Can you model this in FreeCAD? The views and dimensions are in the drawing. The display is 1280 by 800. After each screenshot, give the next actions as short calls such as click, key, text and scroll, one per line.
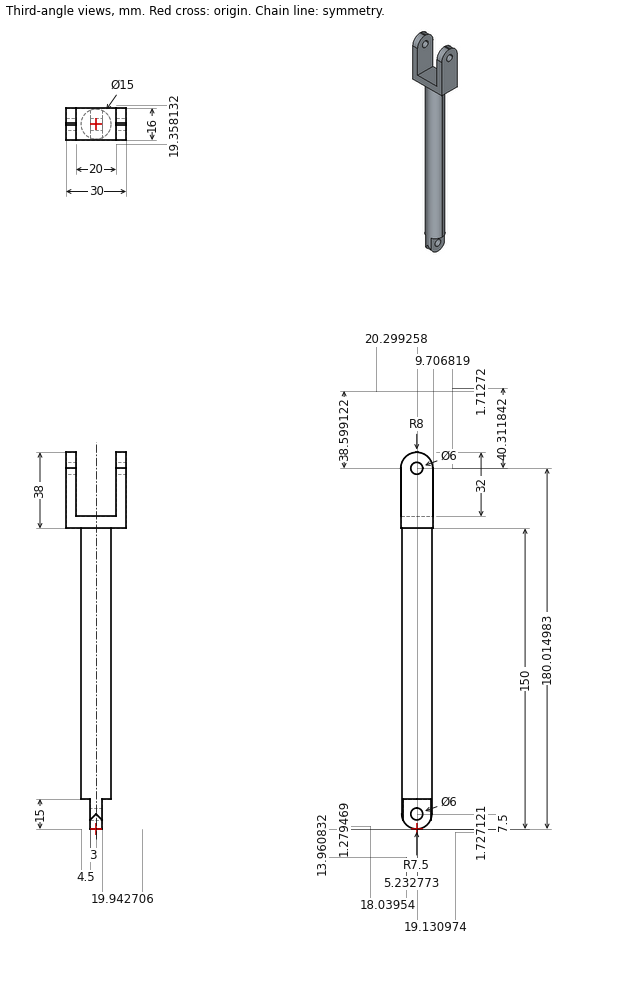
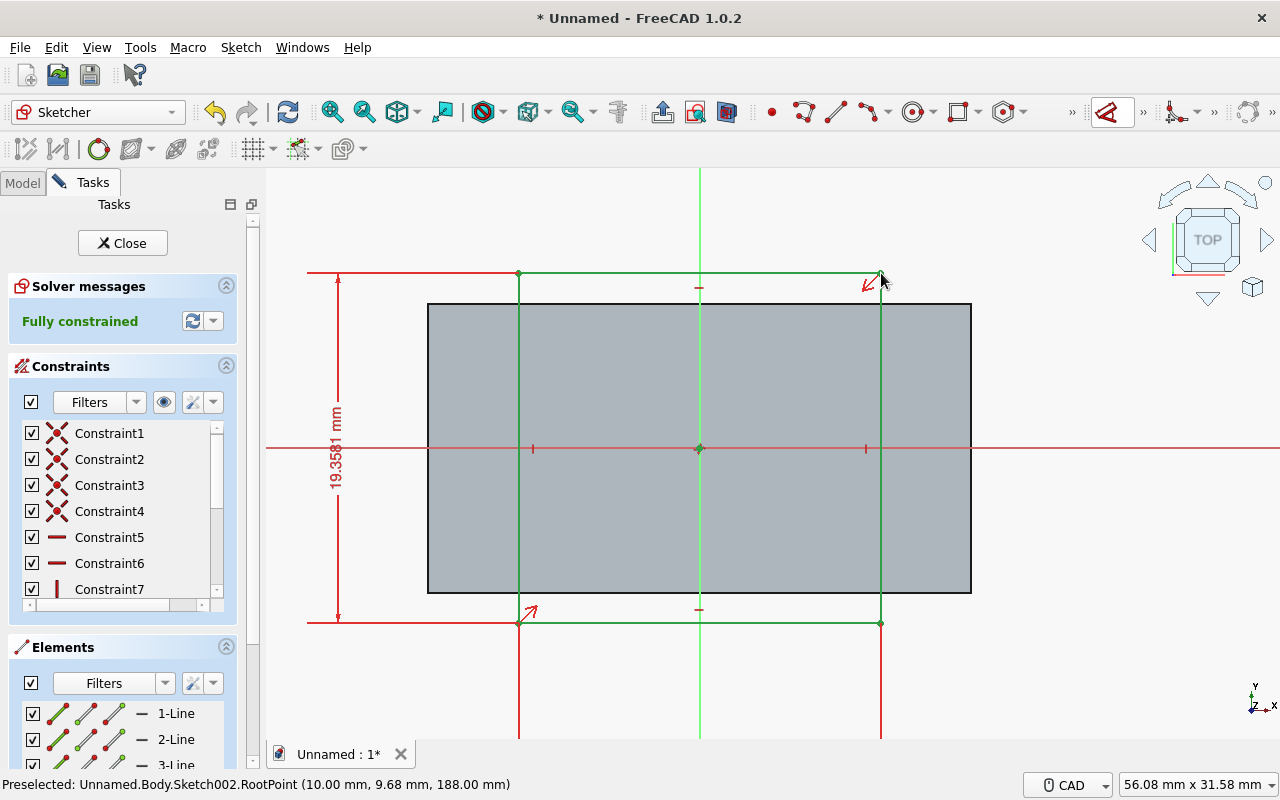
click(123, 243)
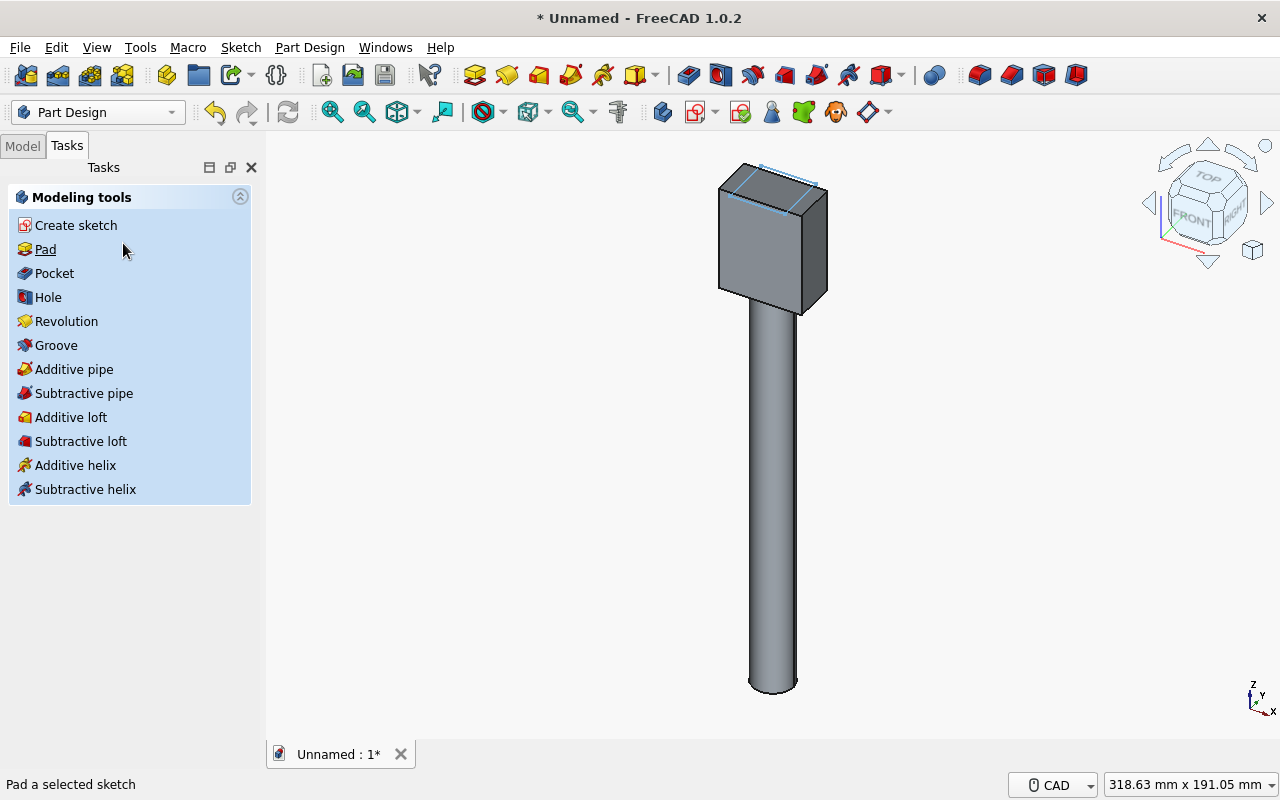
click(690, 76)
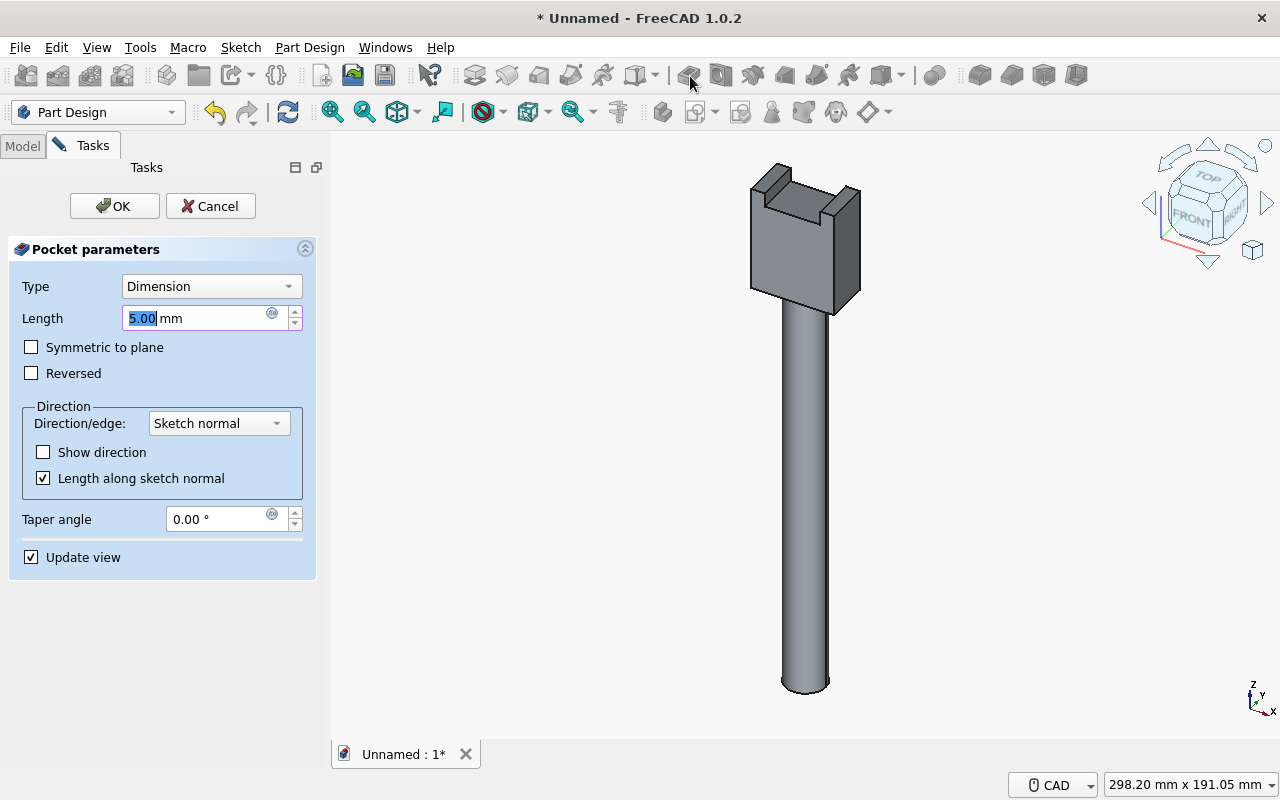
text(32)
key(Tab)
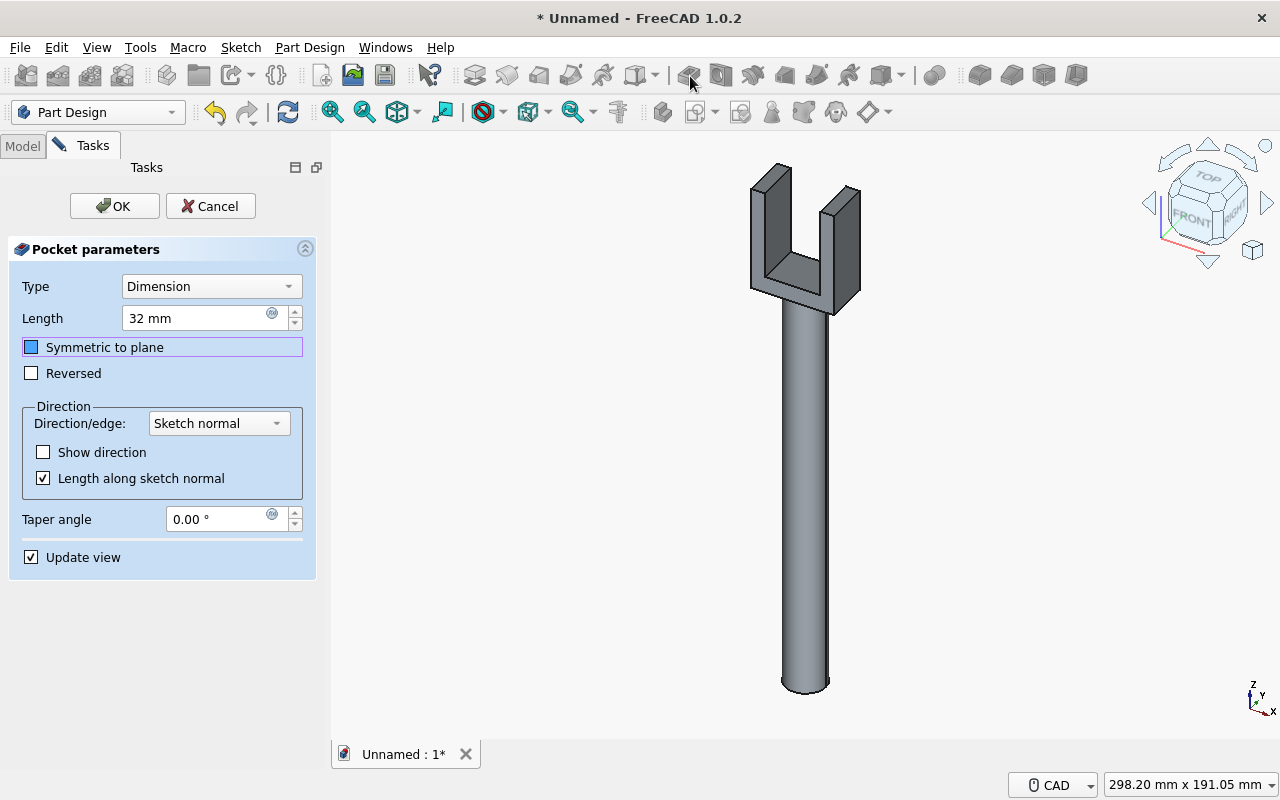
click(115, 206)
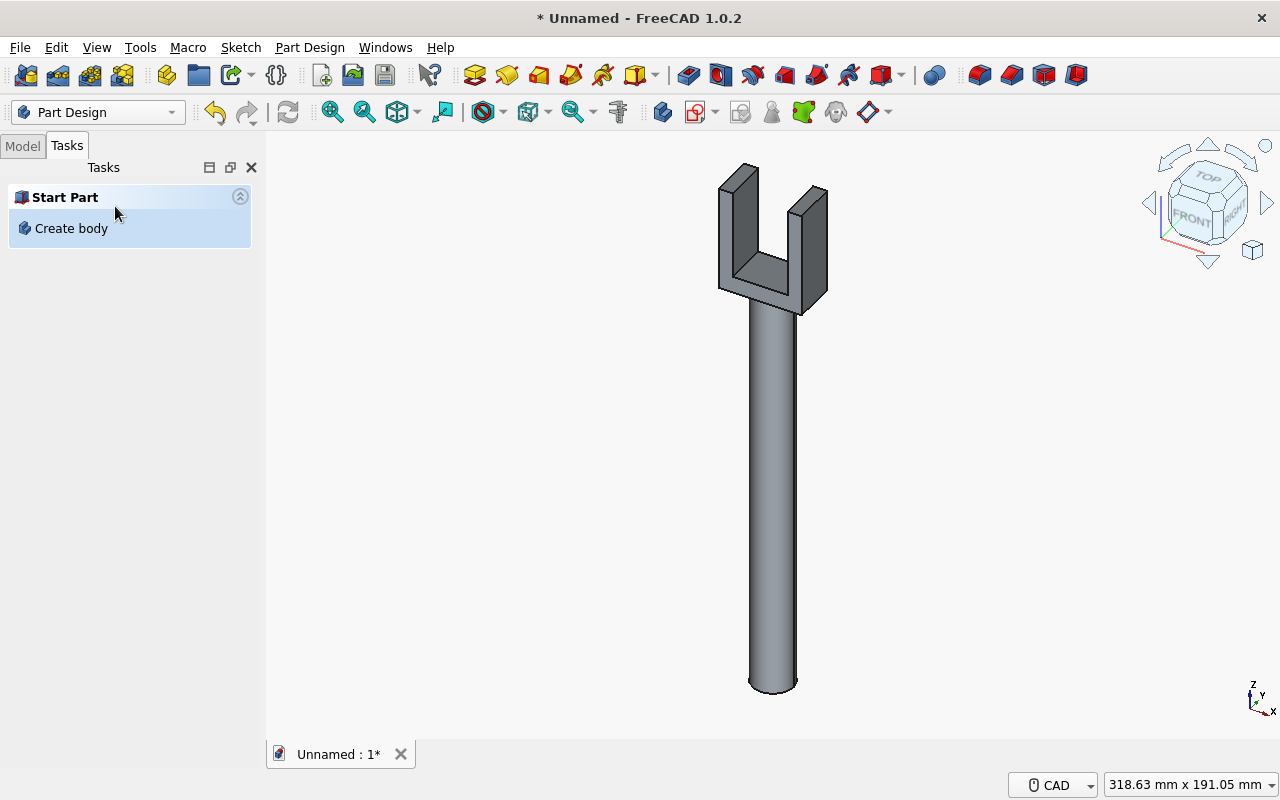
click(814, 224)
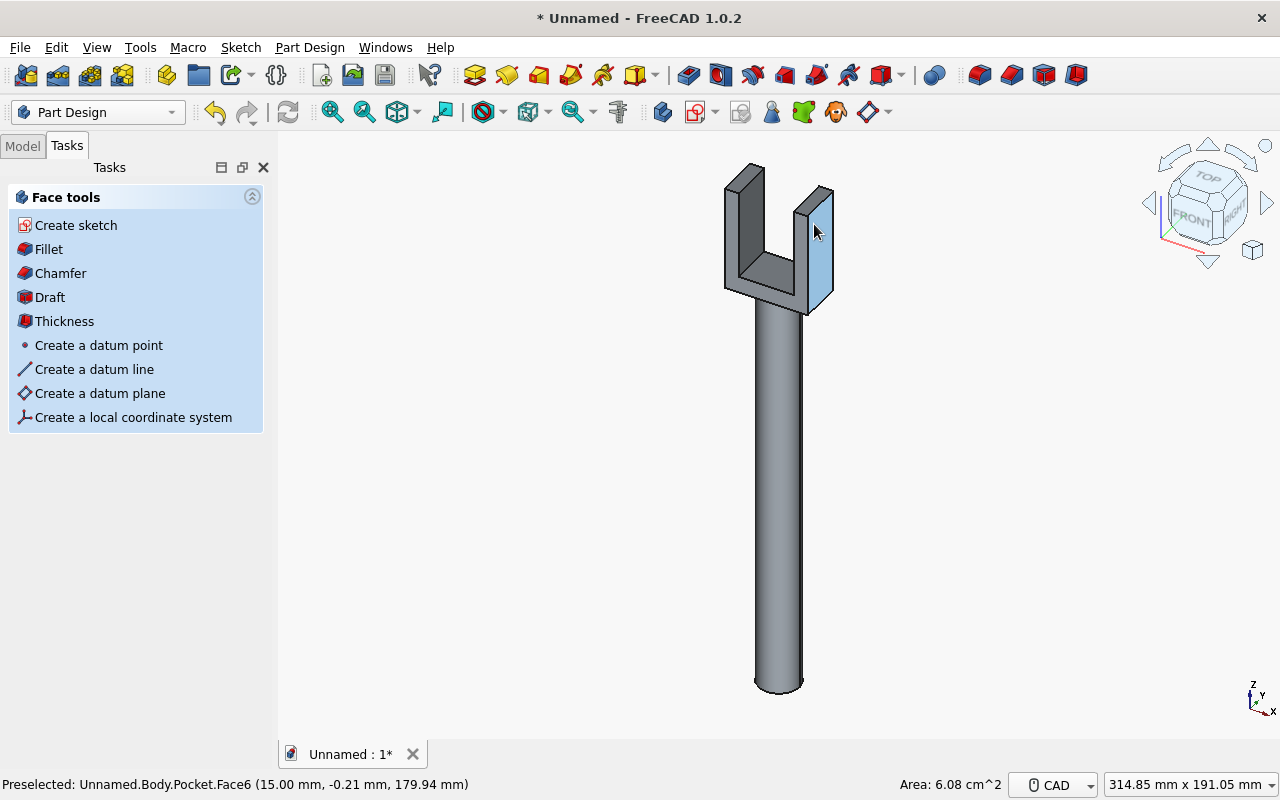
click(696, 112)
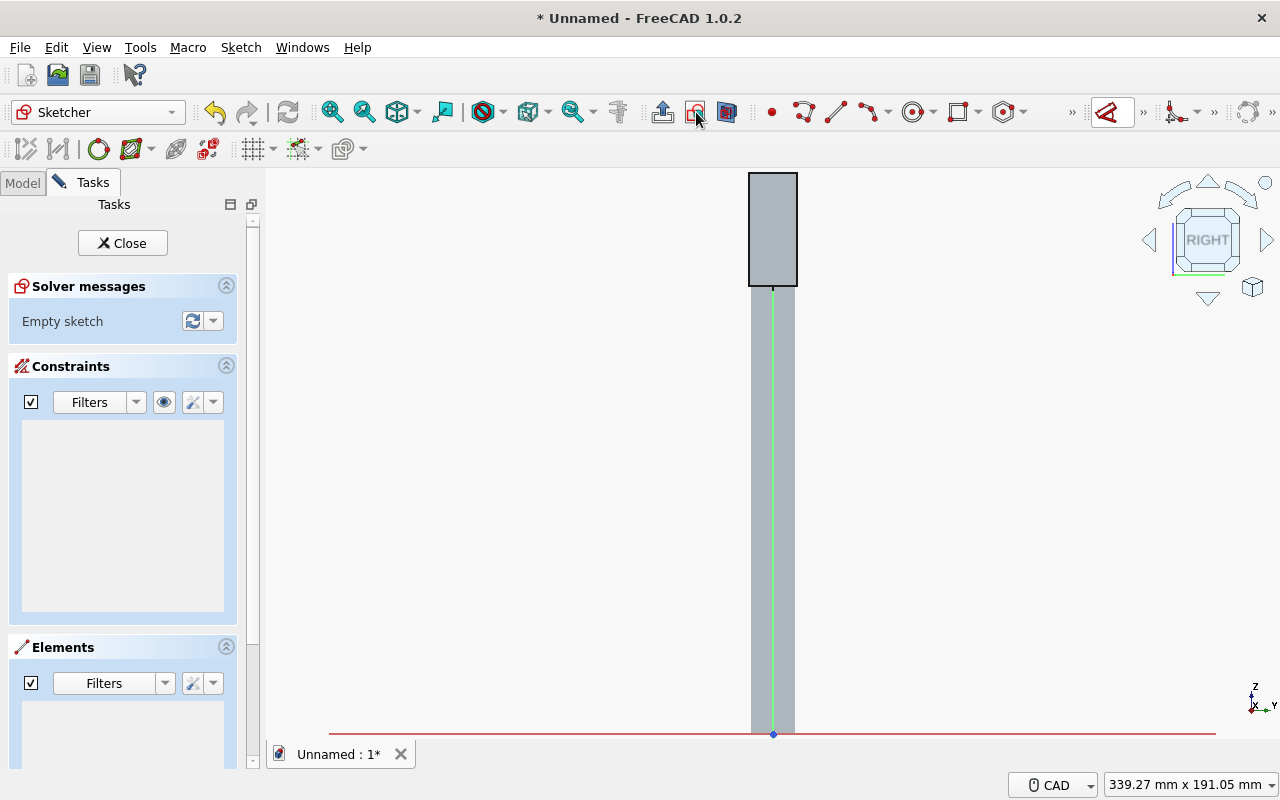
scroll(704, 454, down, 5)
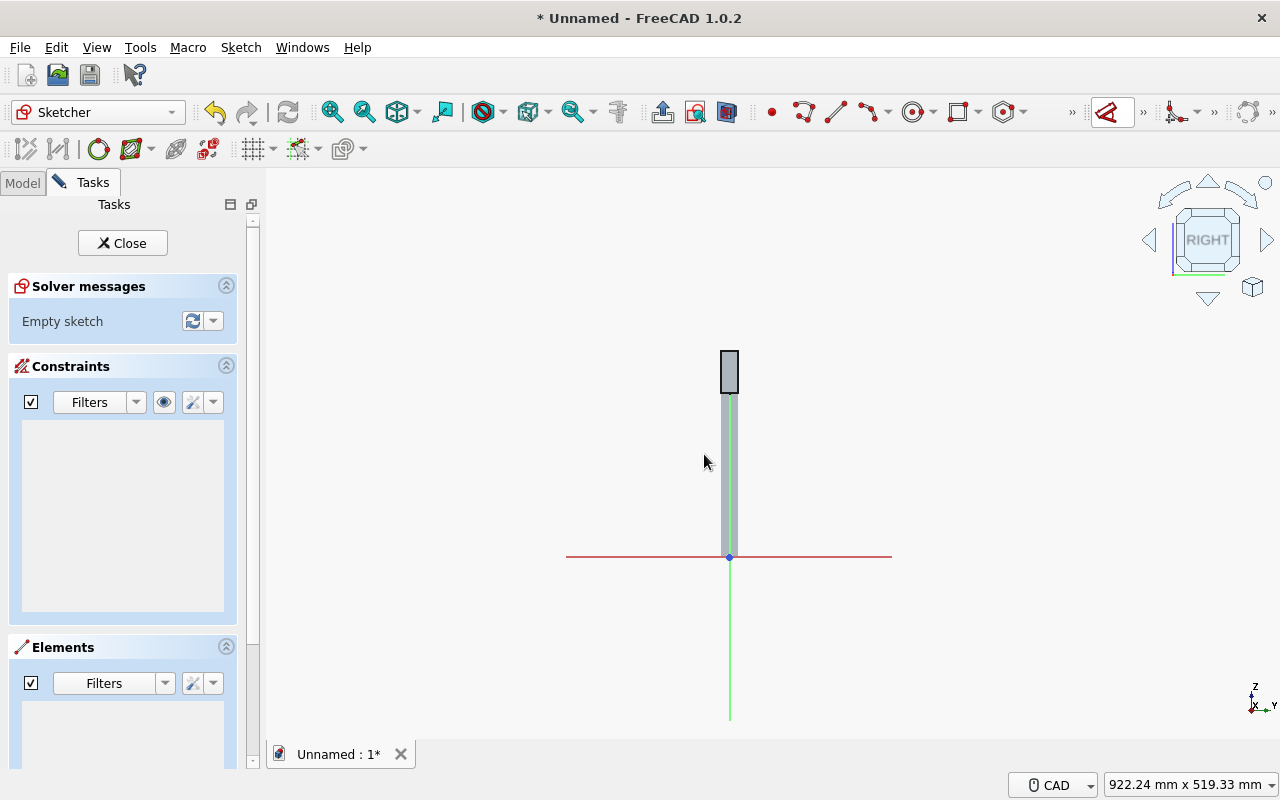
scroll(732, 321, up, 10)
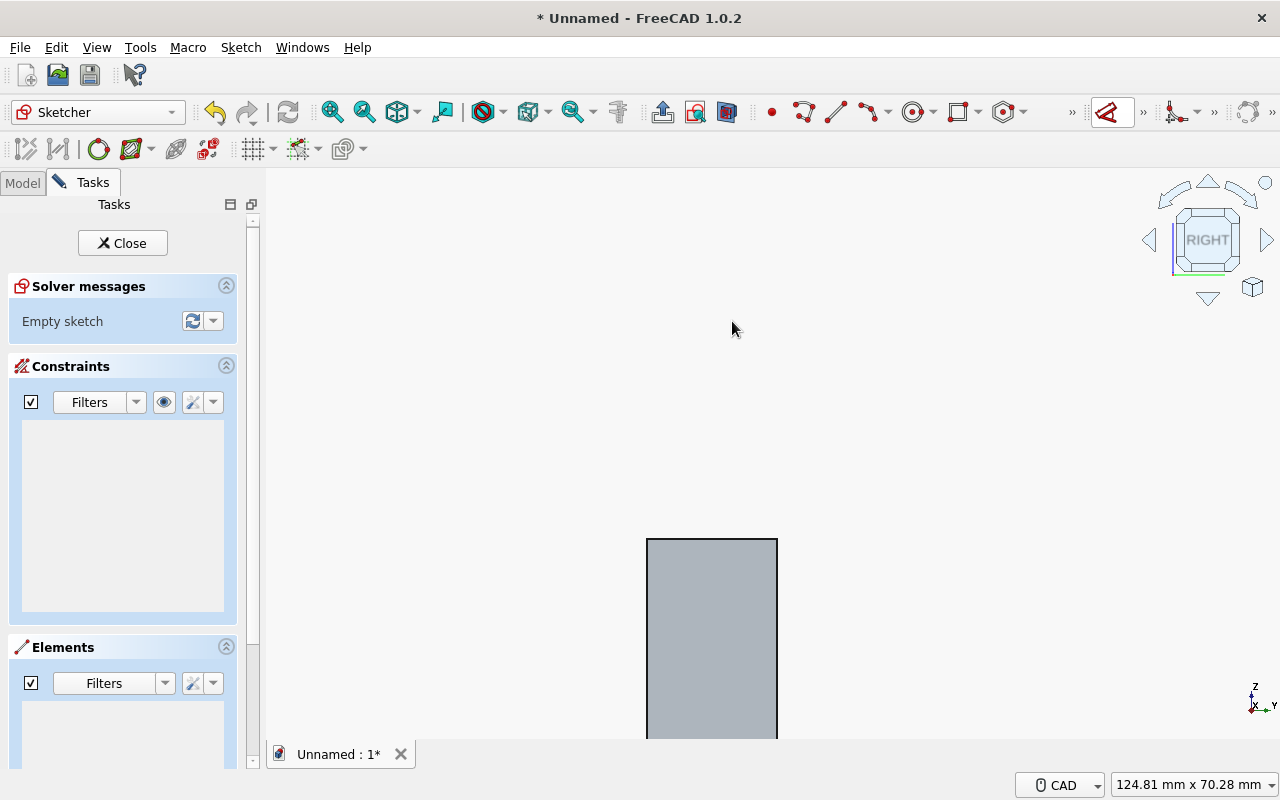
key(g)
key(m)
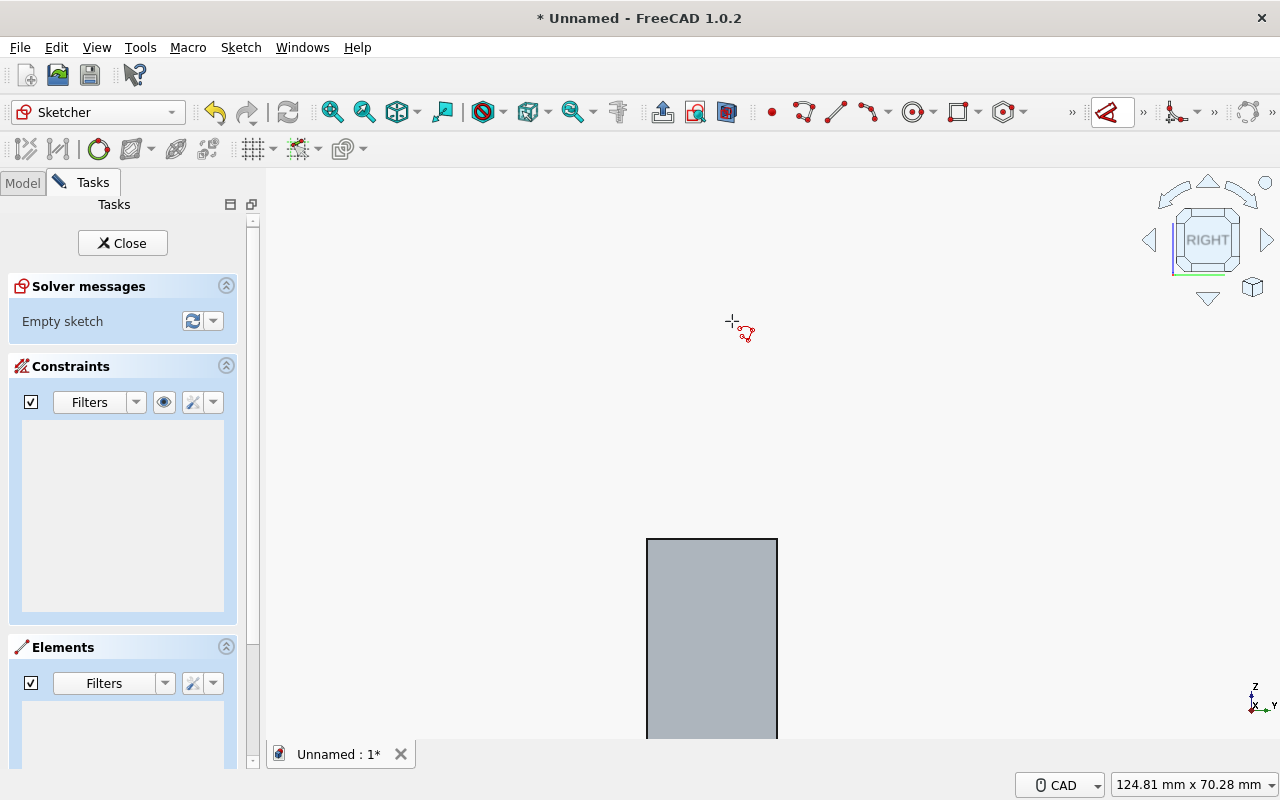
click(777, 604)
click(856, 604)
click(856, 277)
click(547, 292)
click(647, 604)
right_click(647, 604)